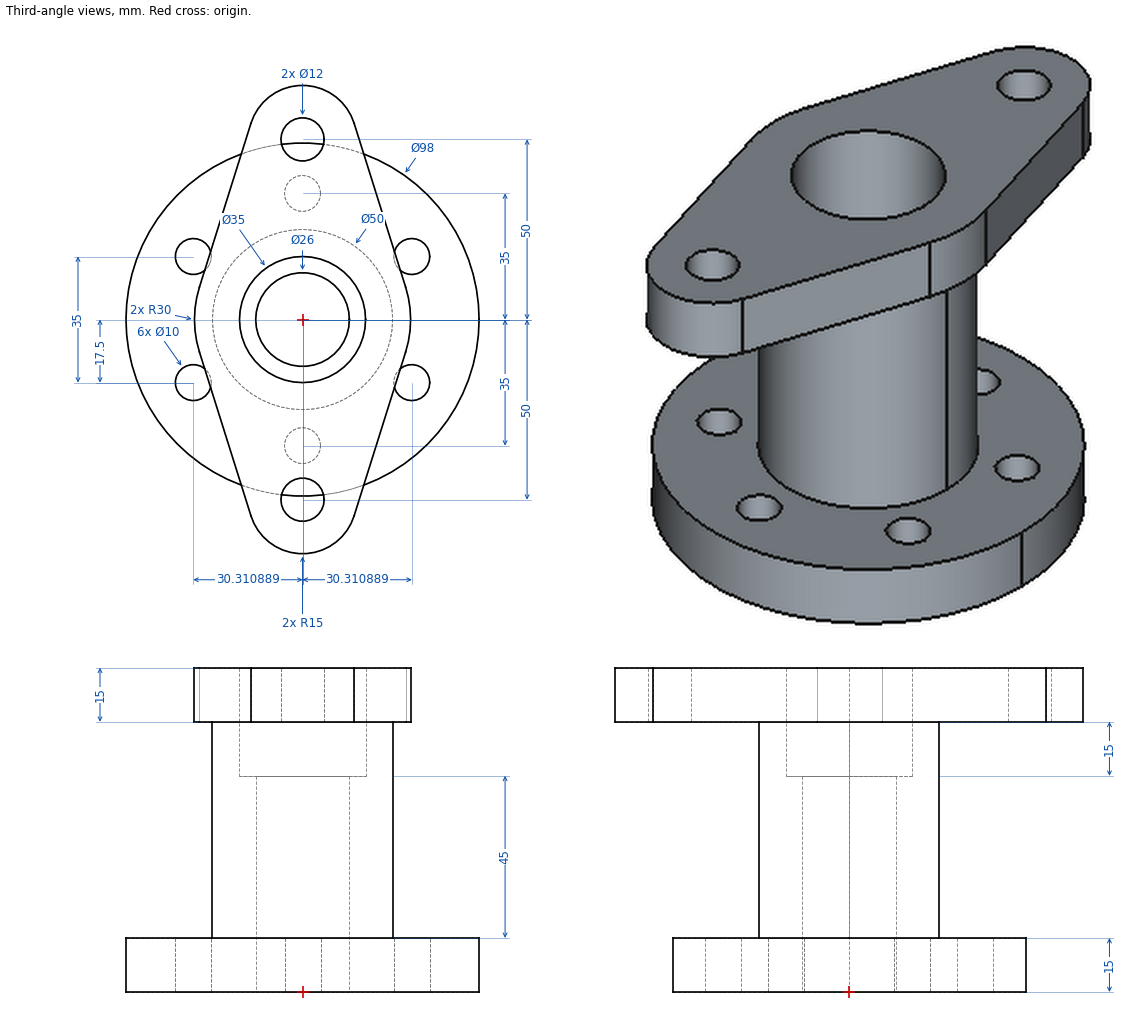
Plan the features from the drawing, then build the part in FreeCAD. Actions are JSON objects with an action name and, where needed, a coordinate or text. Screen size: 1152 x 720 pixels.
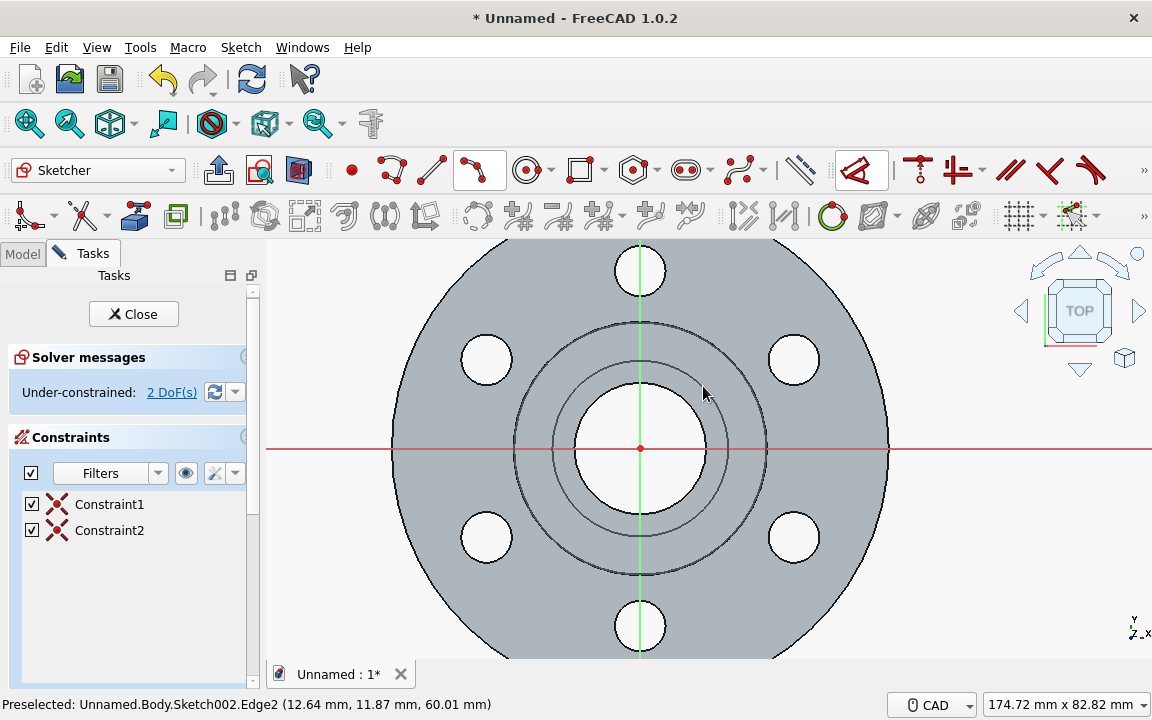
{"action": "left_click", "coordinate": [729, 359]}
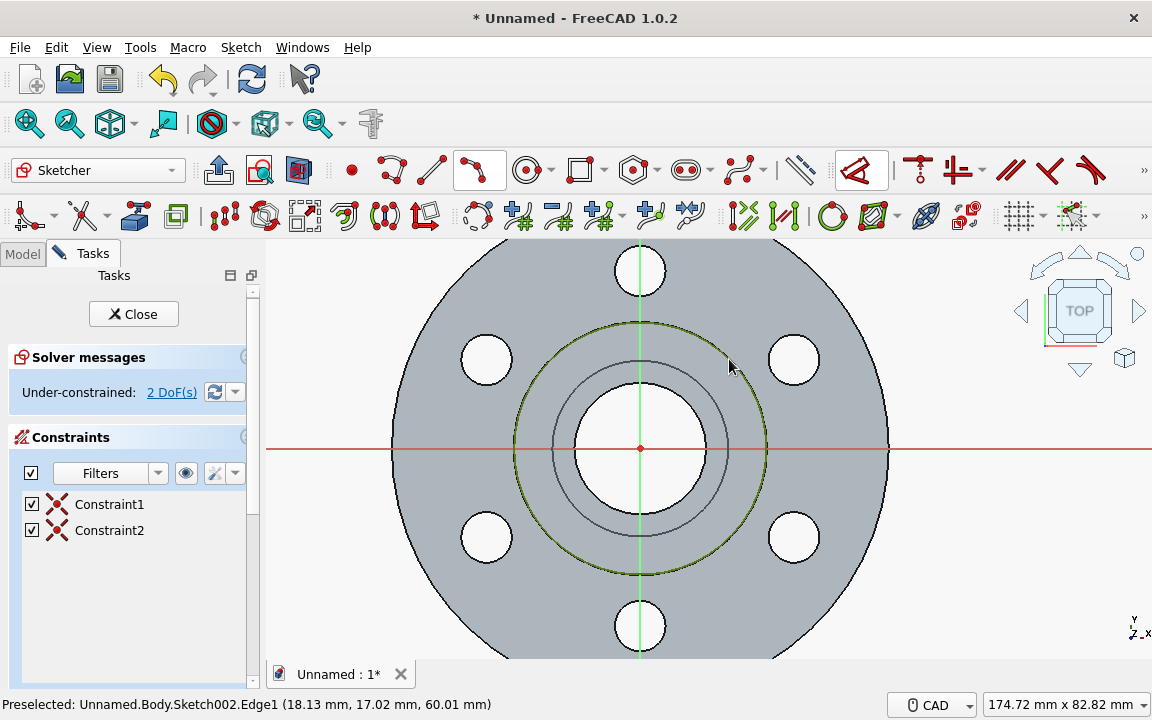
{"action": "key", "text": "k o"}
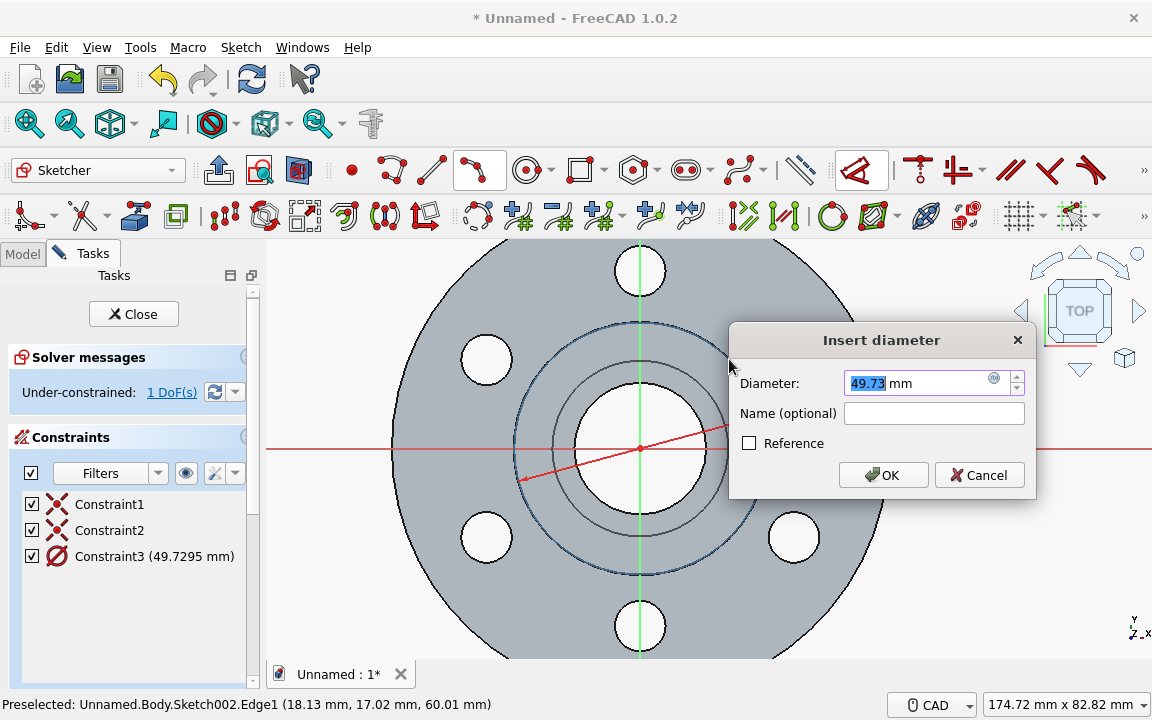
{"action": "type", "text": "50"}
{"action": "key", "text": "Return"}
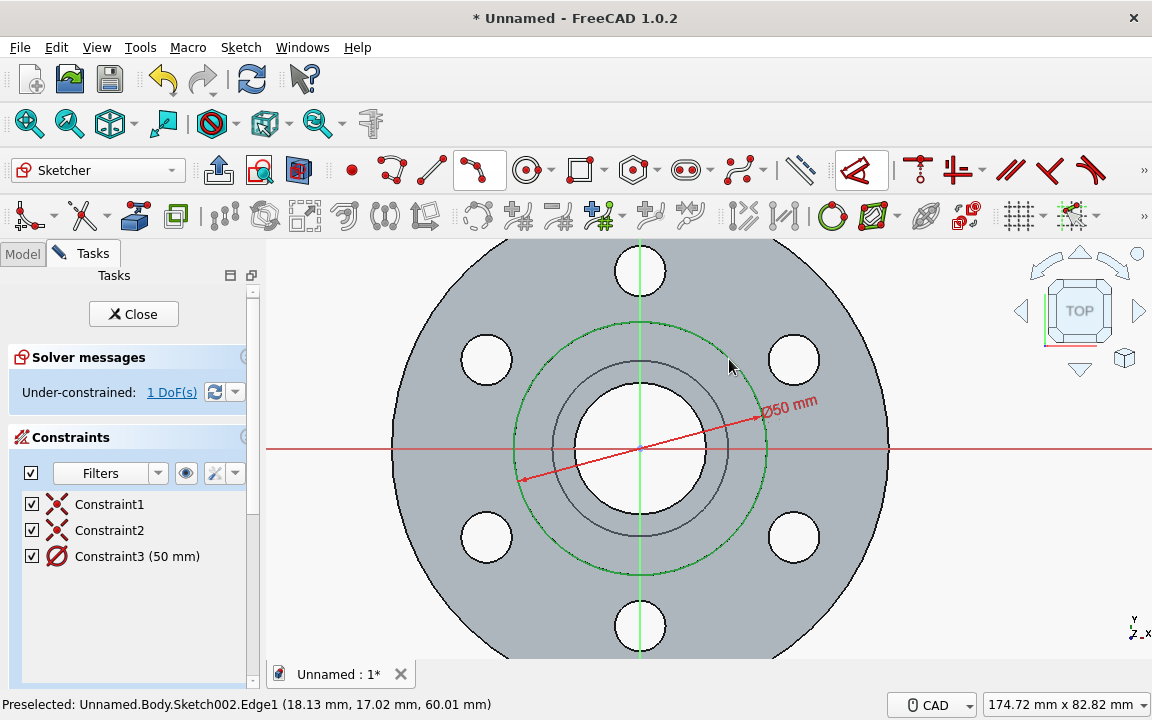
{"action": "left_click", "coordinate": [702, 386]}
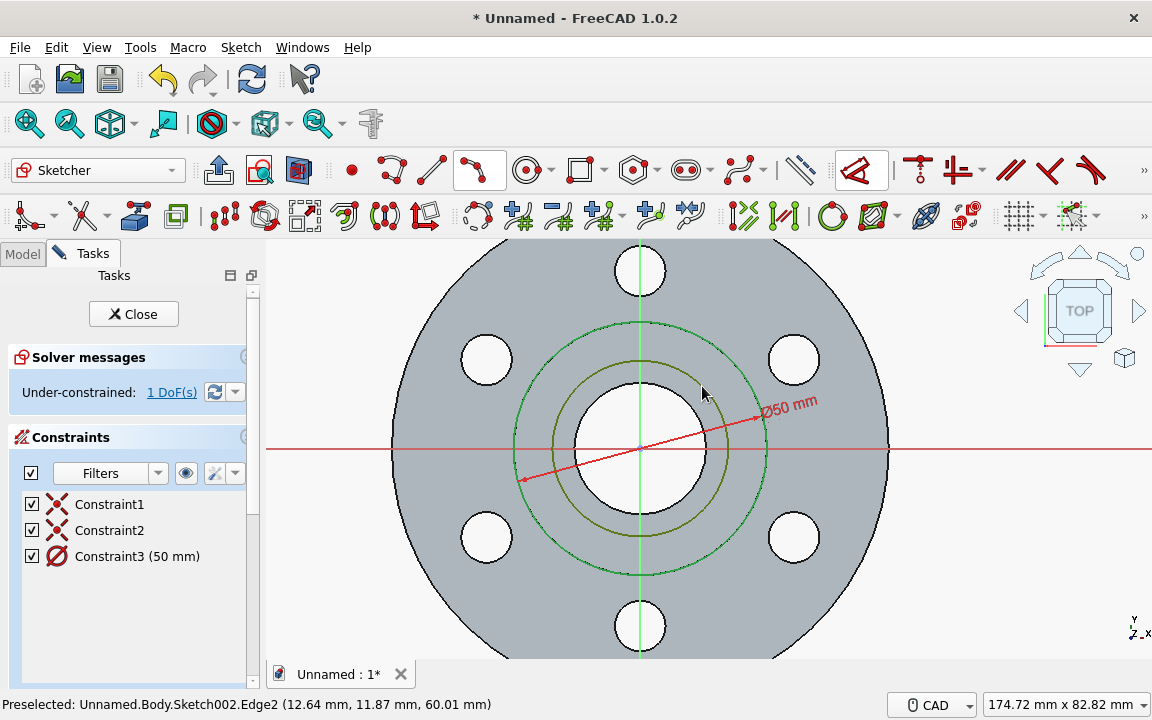
{"action": "key", "text": "k o"}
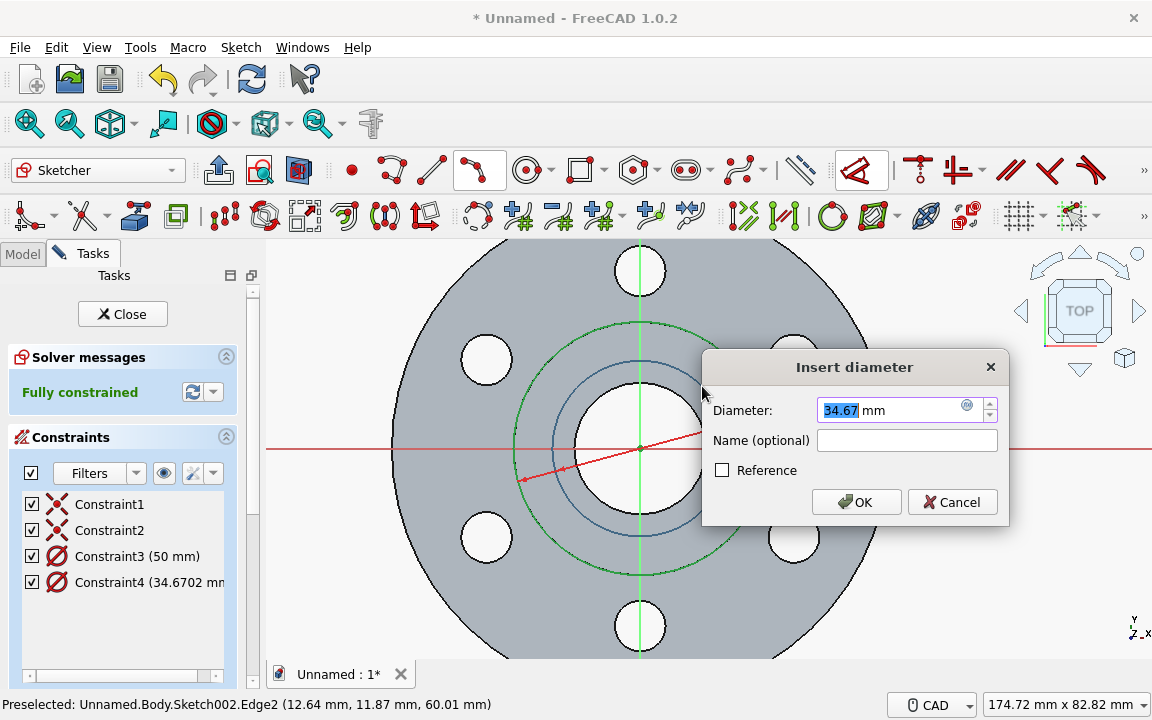
{"action": "type", "text": "35"}
{"action": "key", "text": "Return"}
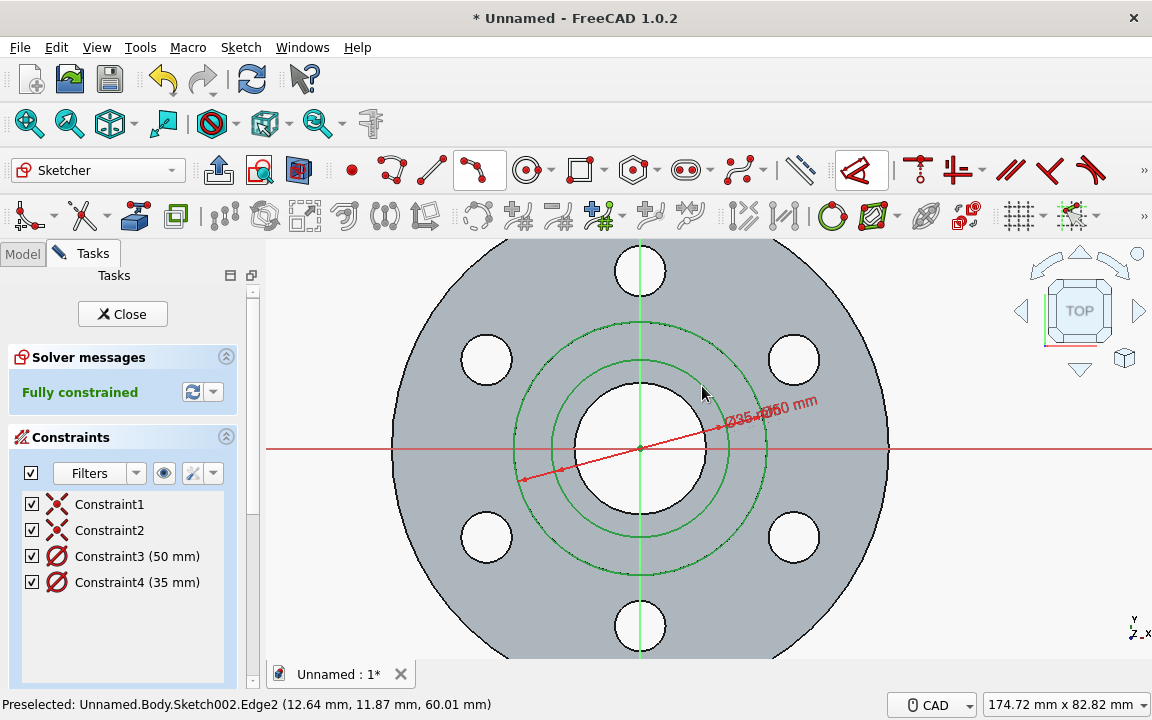
{"action": "left_click", "coordinate": [123, 314]}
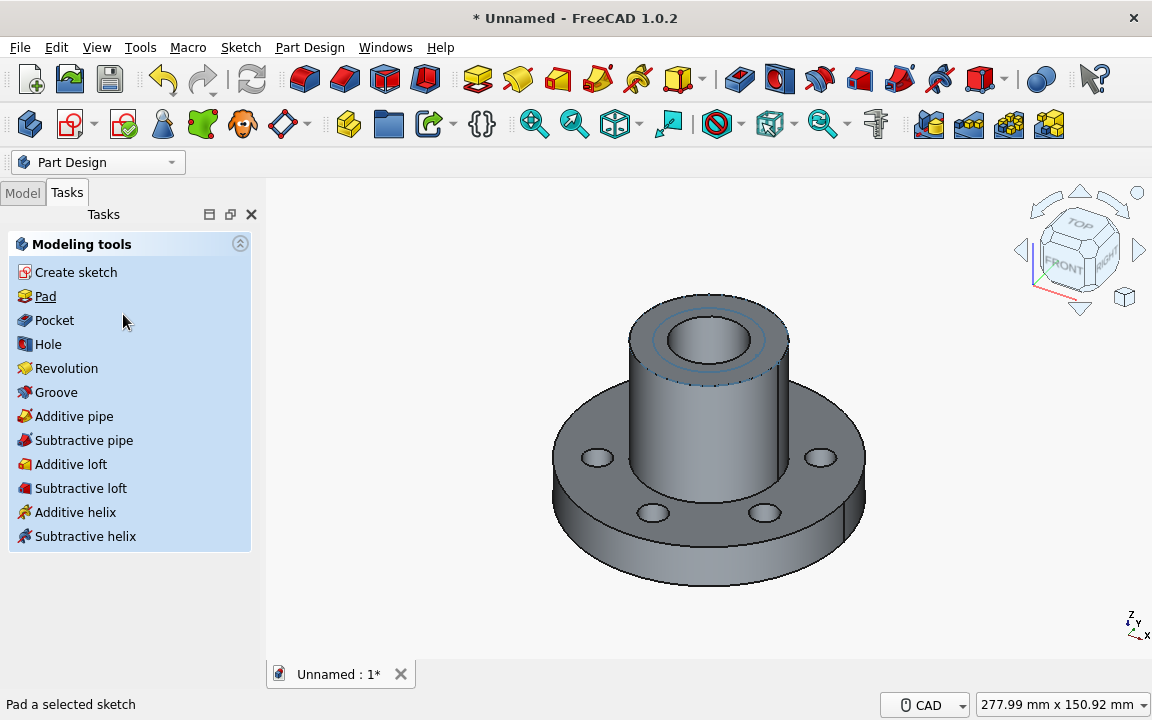
{"action": "left_click", "coordinate": [478, 80]}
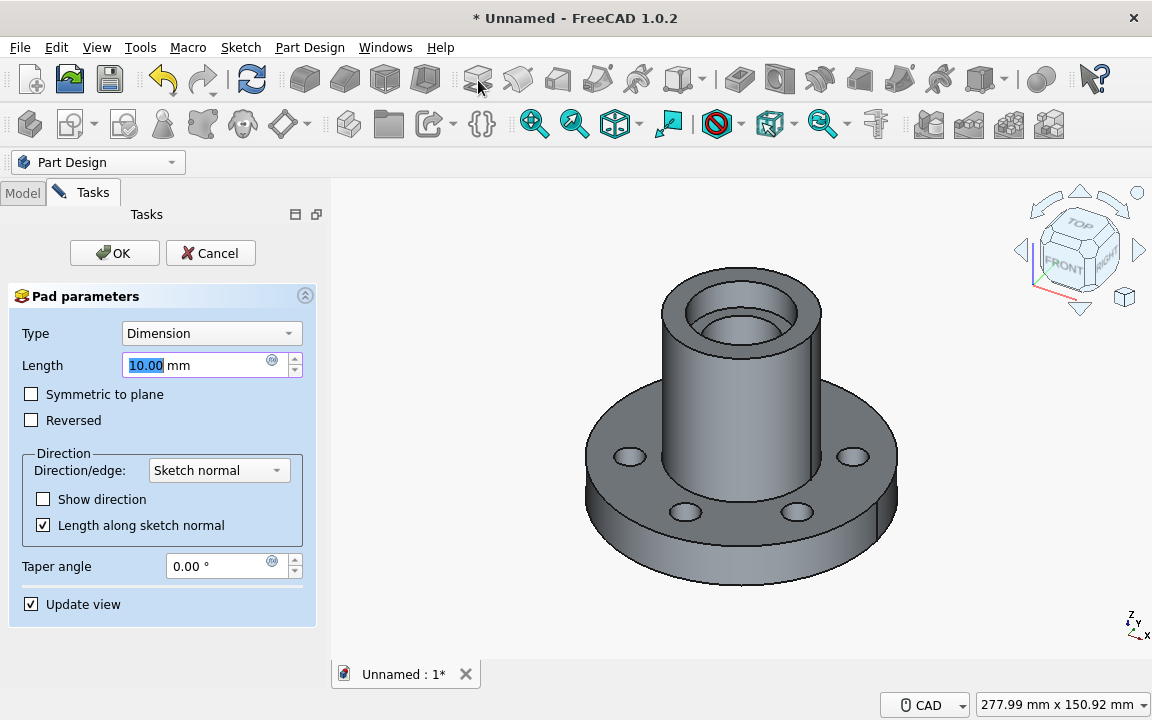
{"action": "type", "text": "15"}
{"action": "key", "text": "Tab"}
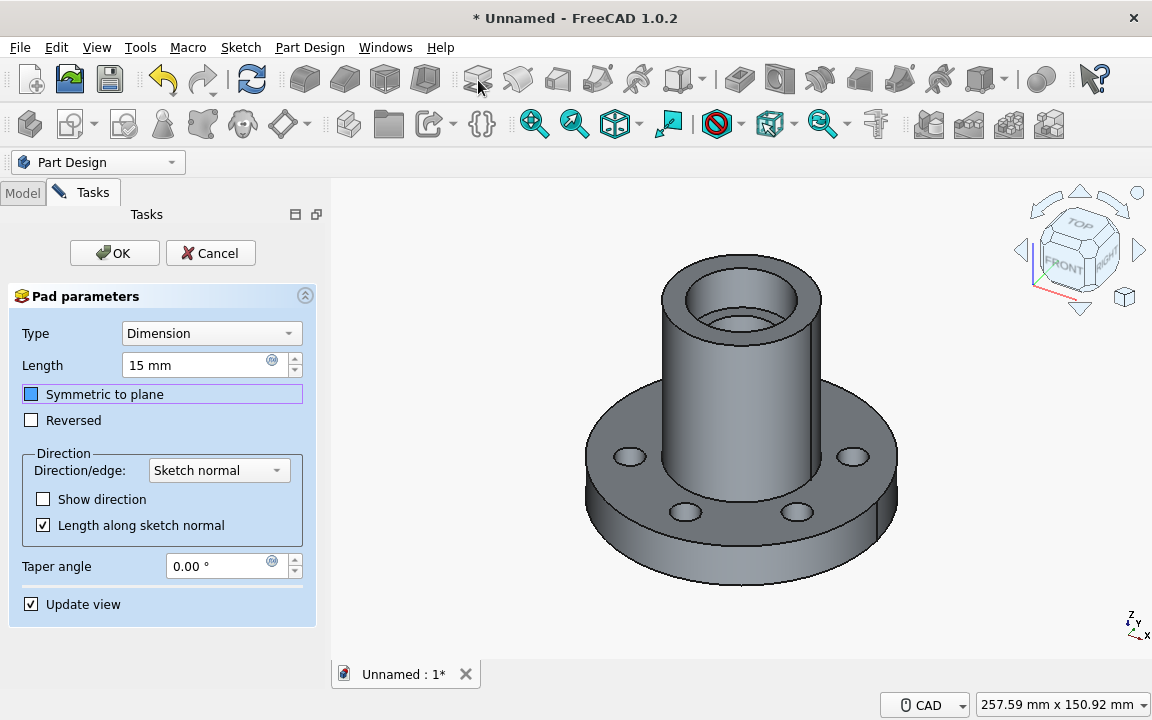
{"action": "left_click", "coordinate": [115, 253]}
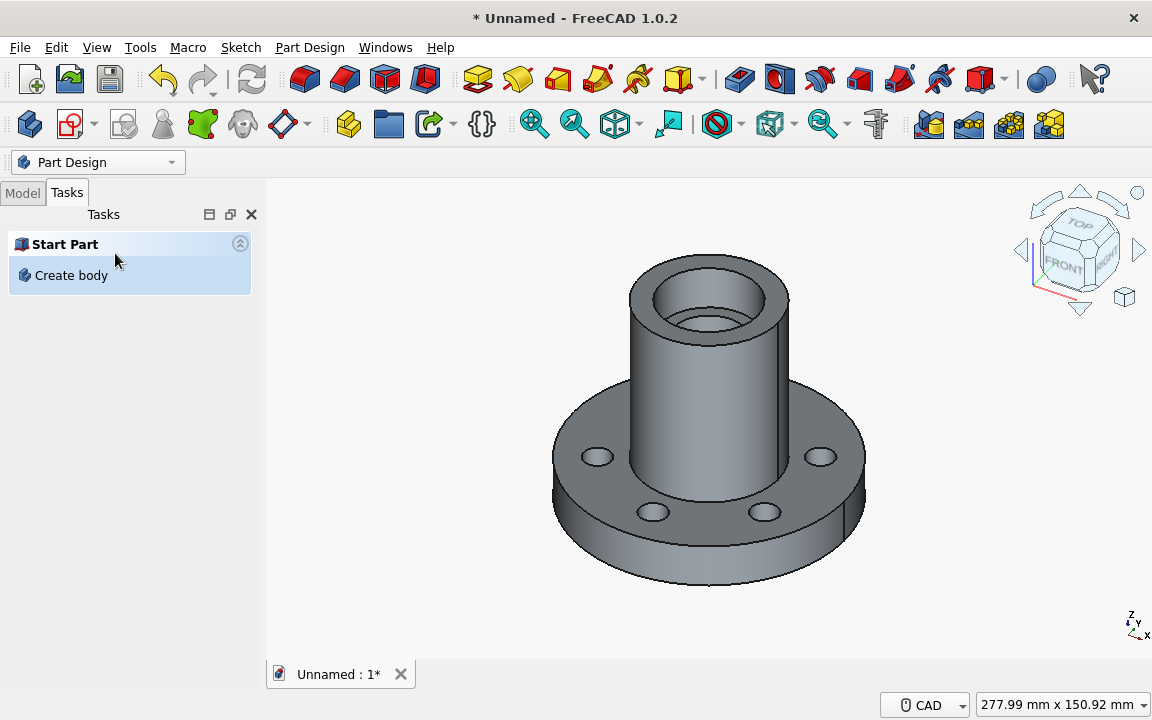
{"action": "left_click", "coordinate": [536, 124]}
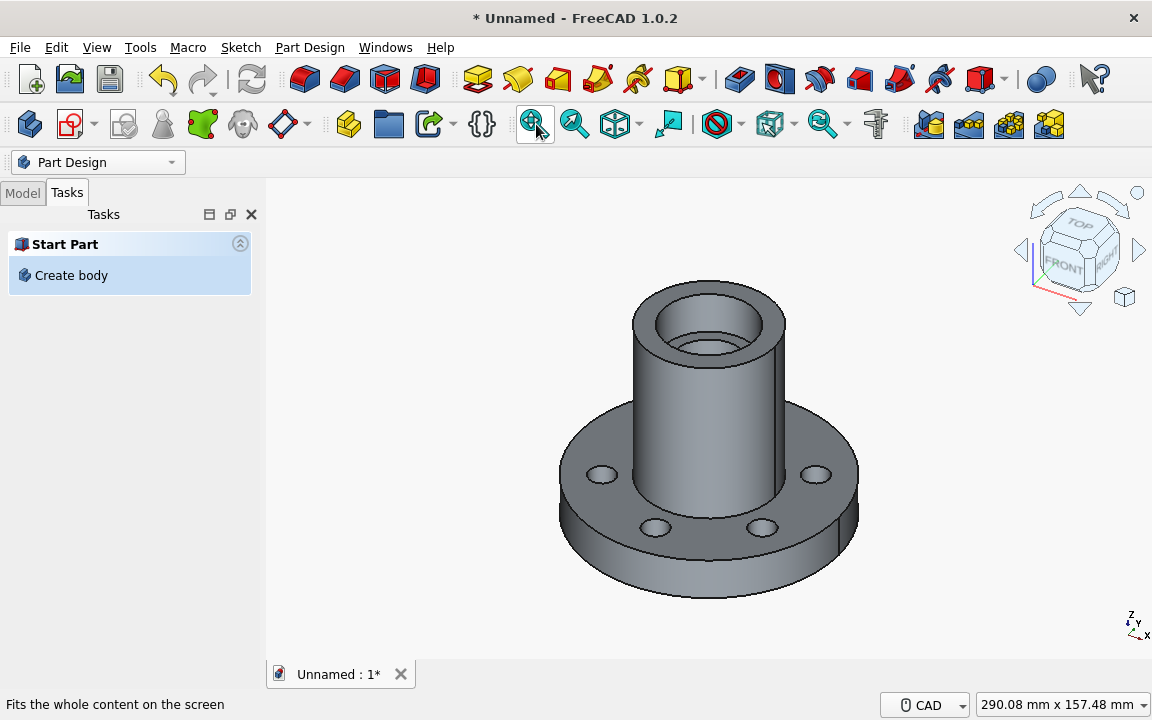
{"action": "left_click", "coordinate": [652, 305]}